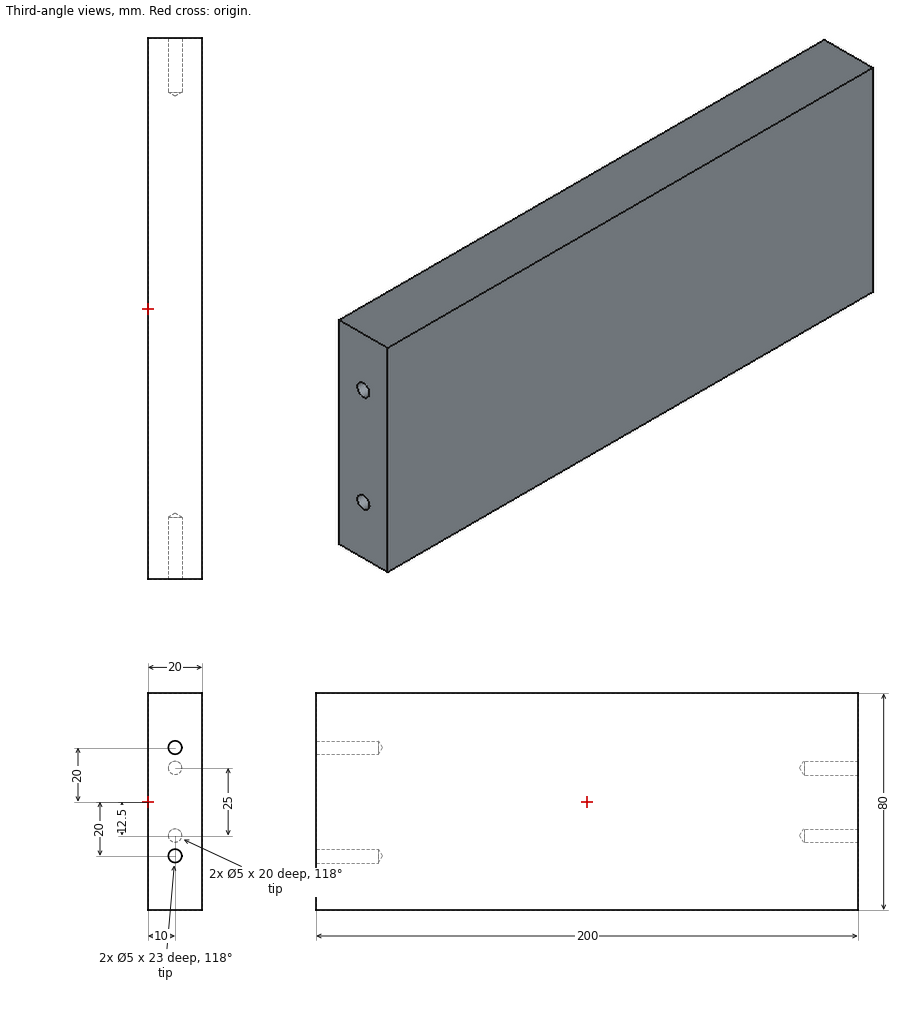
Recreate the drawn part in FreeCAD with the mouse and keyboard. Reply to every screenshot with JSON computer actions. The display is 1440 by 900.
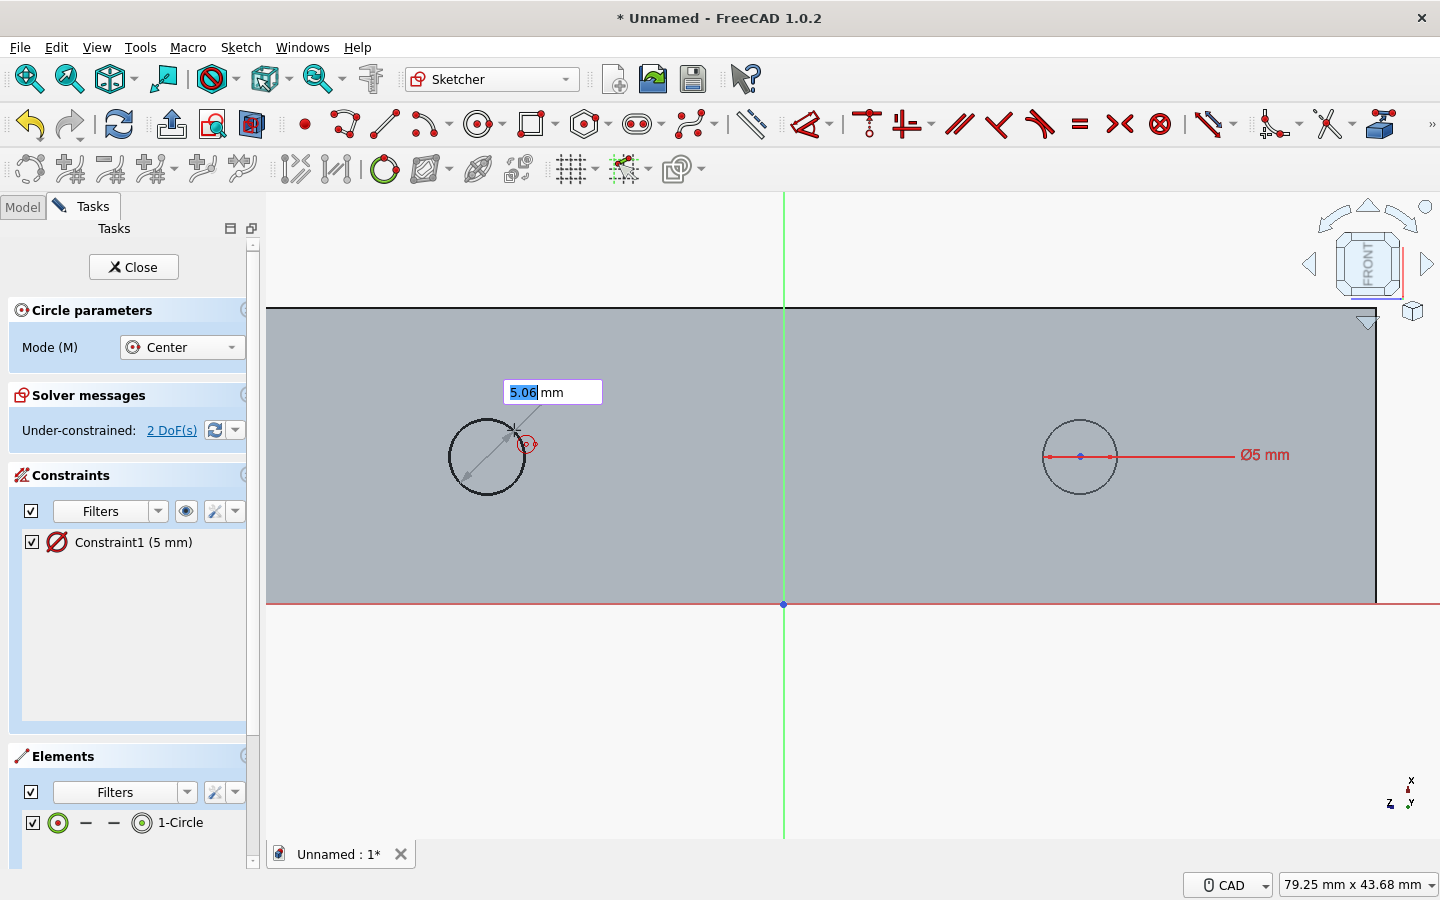
{"action": "type", "text": "5"}
{"action": "key", "text": "Return"}
{"action": "key", "text": "Escape"}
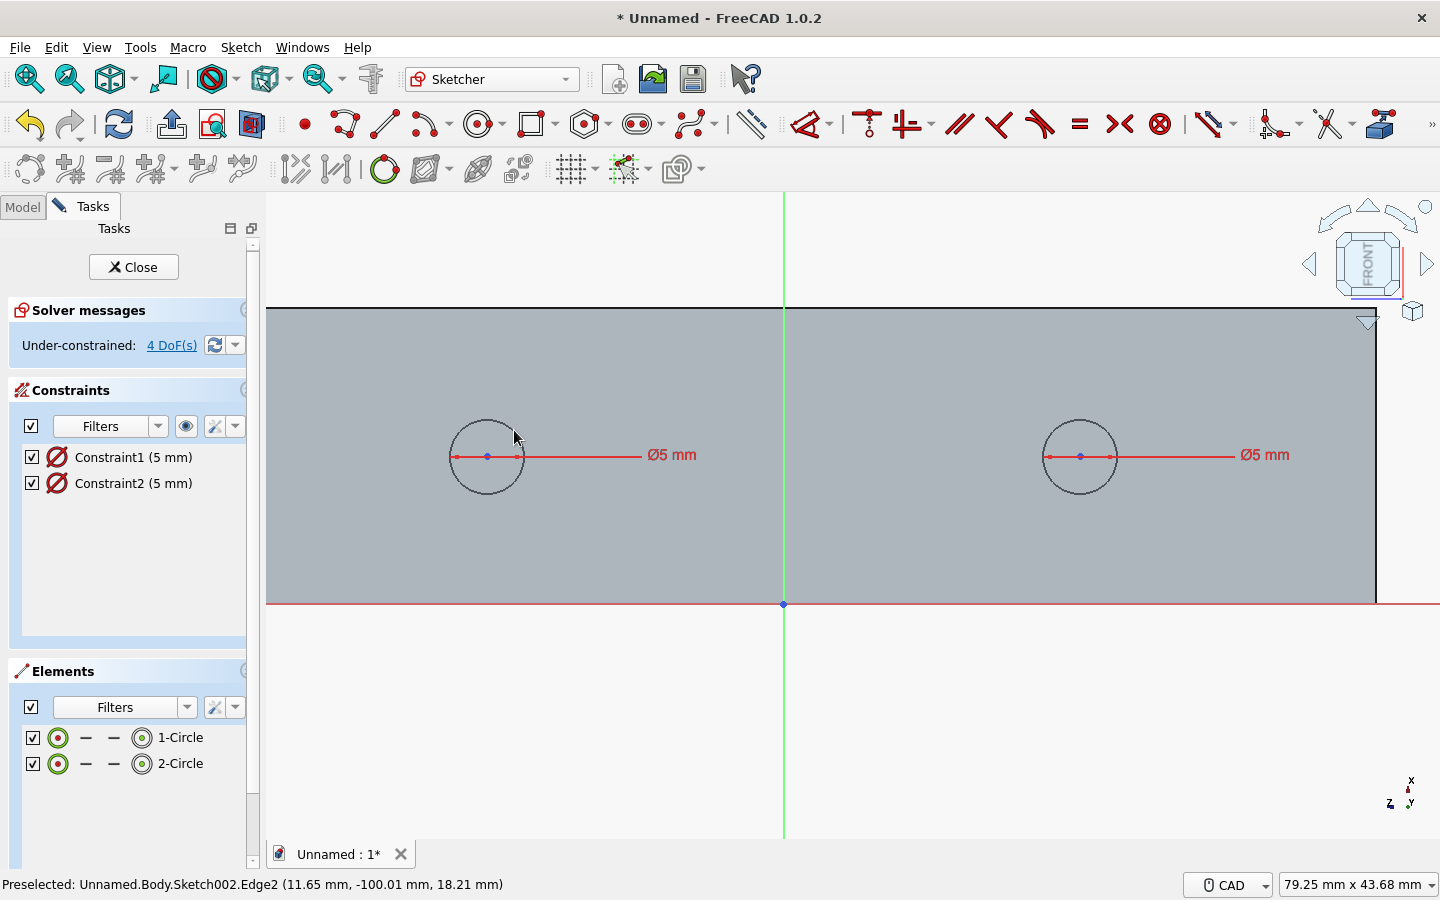
{"action": "left_click", "coordinate": [1080, 457]}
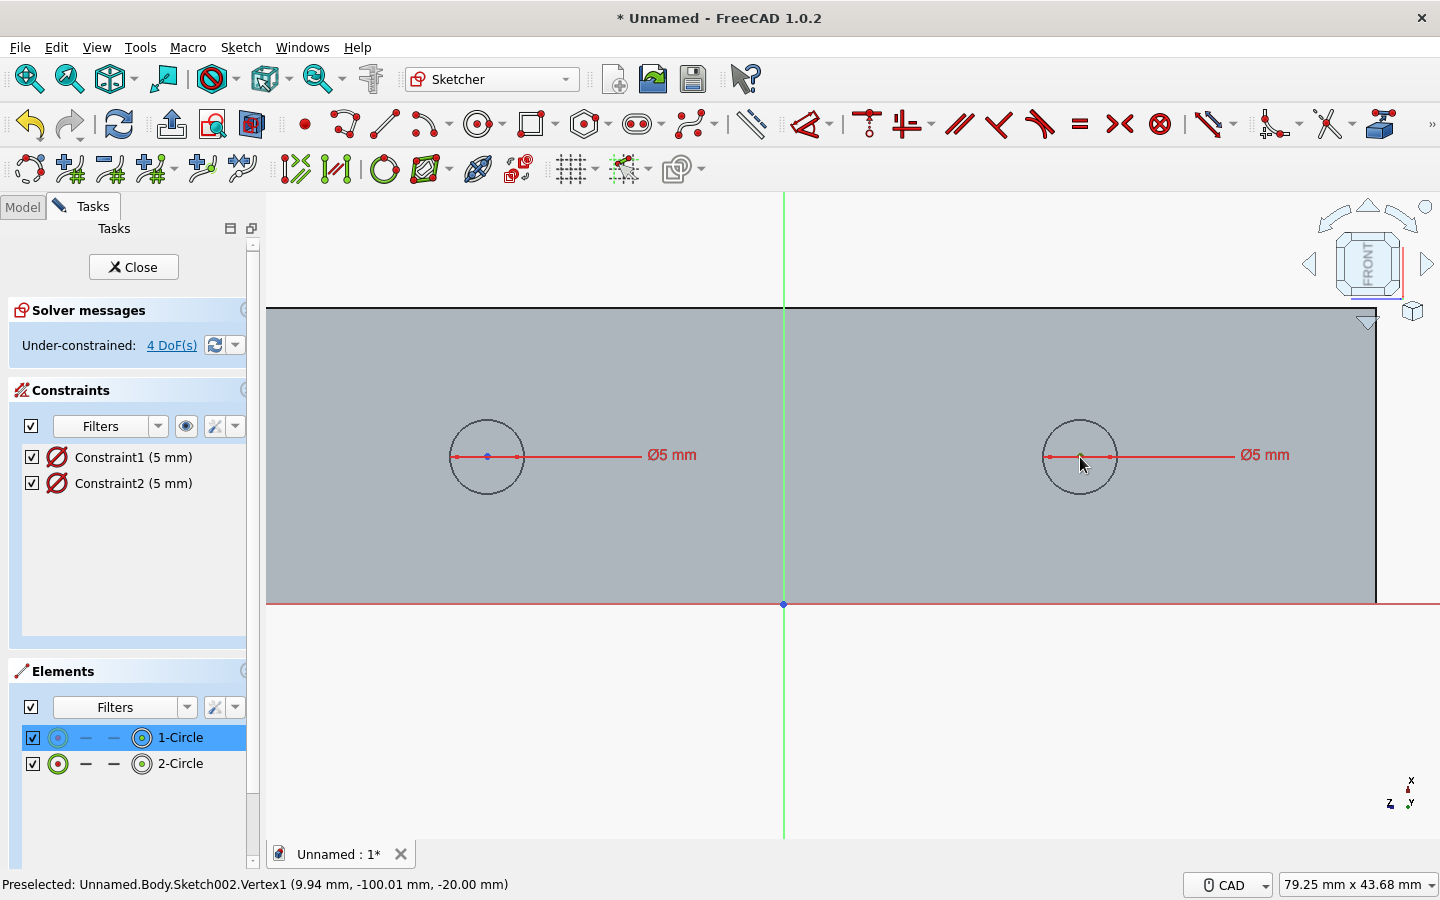
{"action": "left_click", "coordinate": [487, 457]}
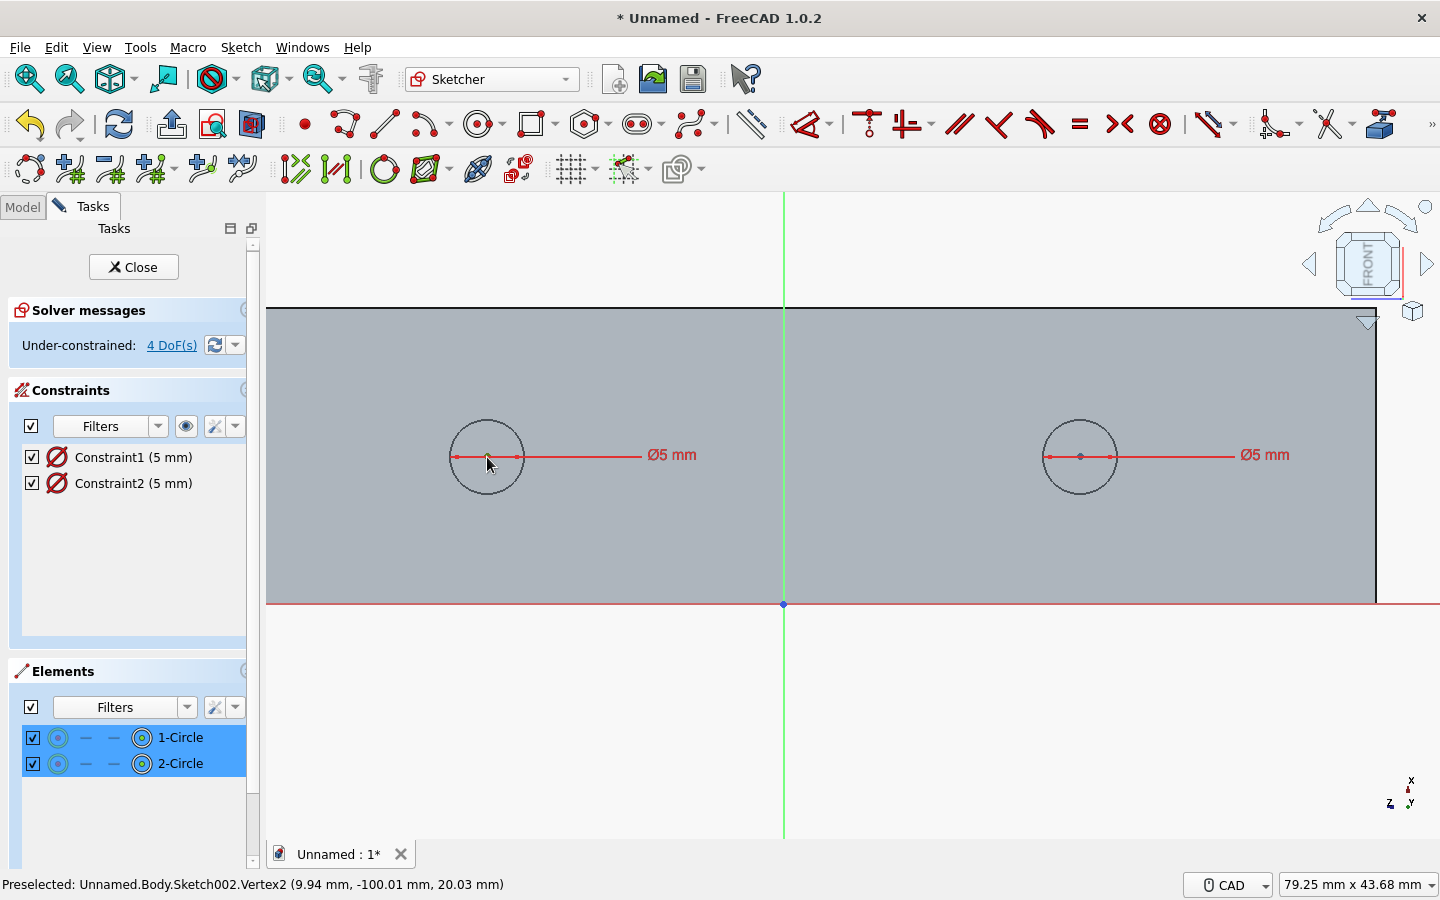
{"action": "key", "text": "h"}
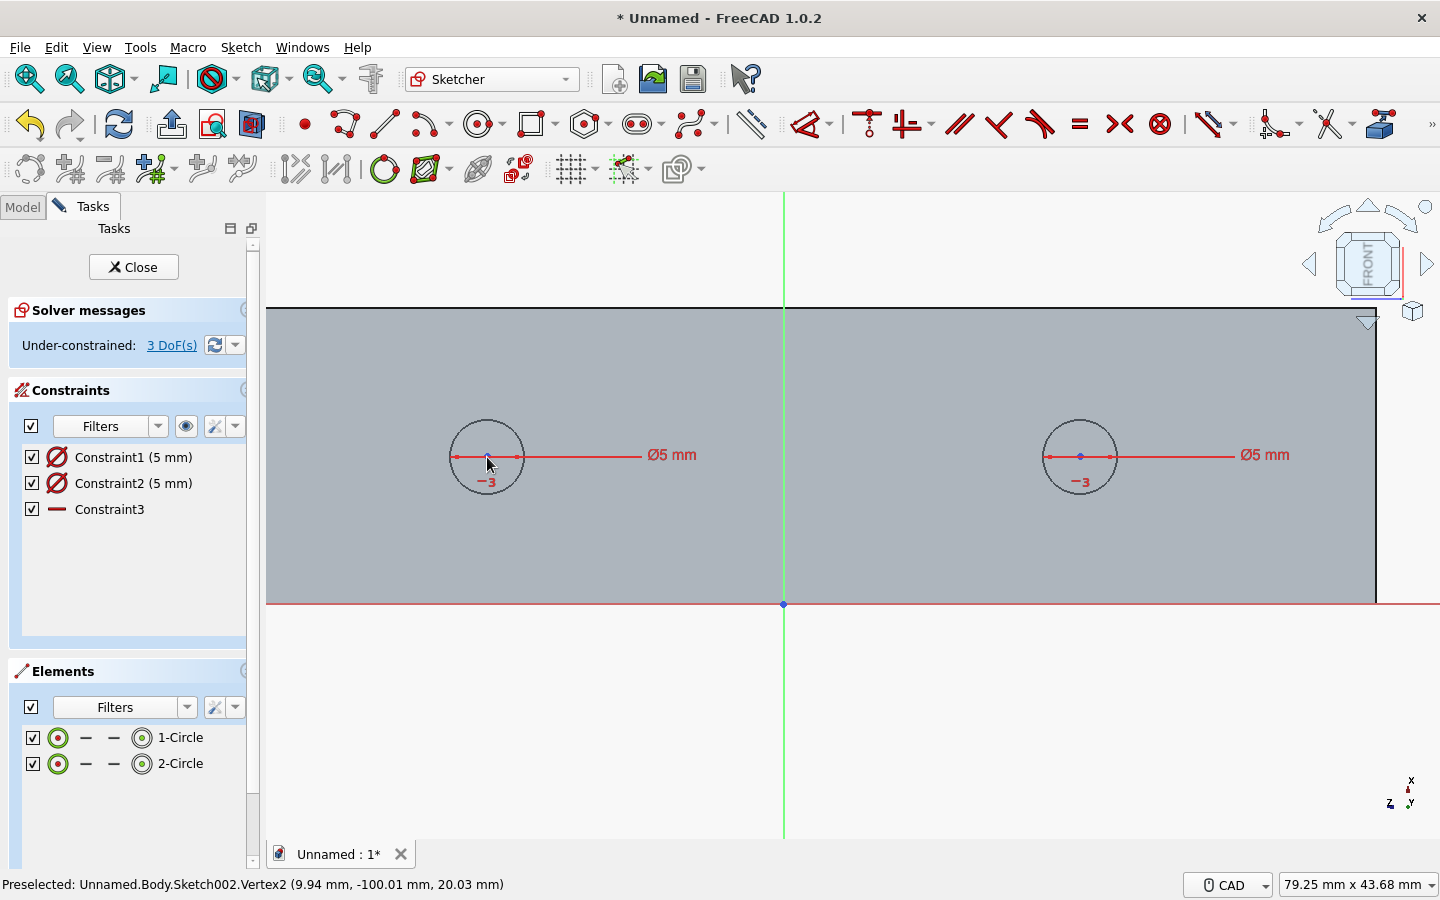
{"action": "left_click", "coordinate": [806, 124]}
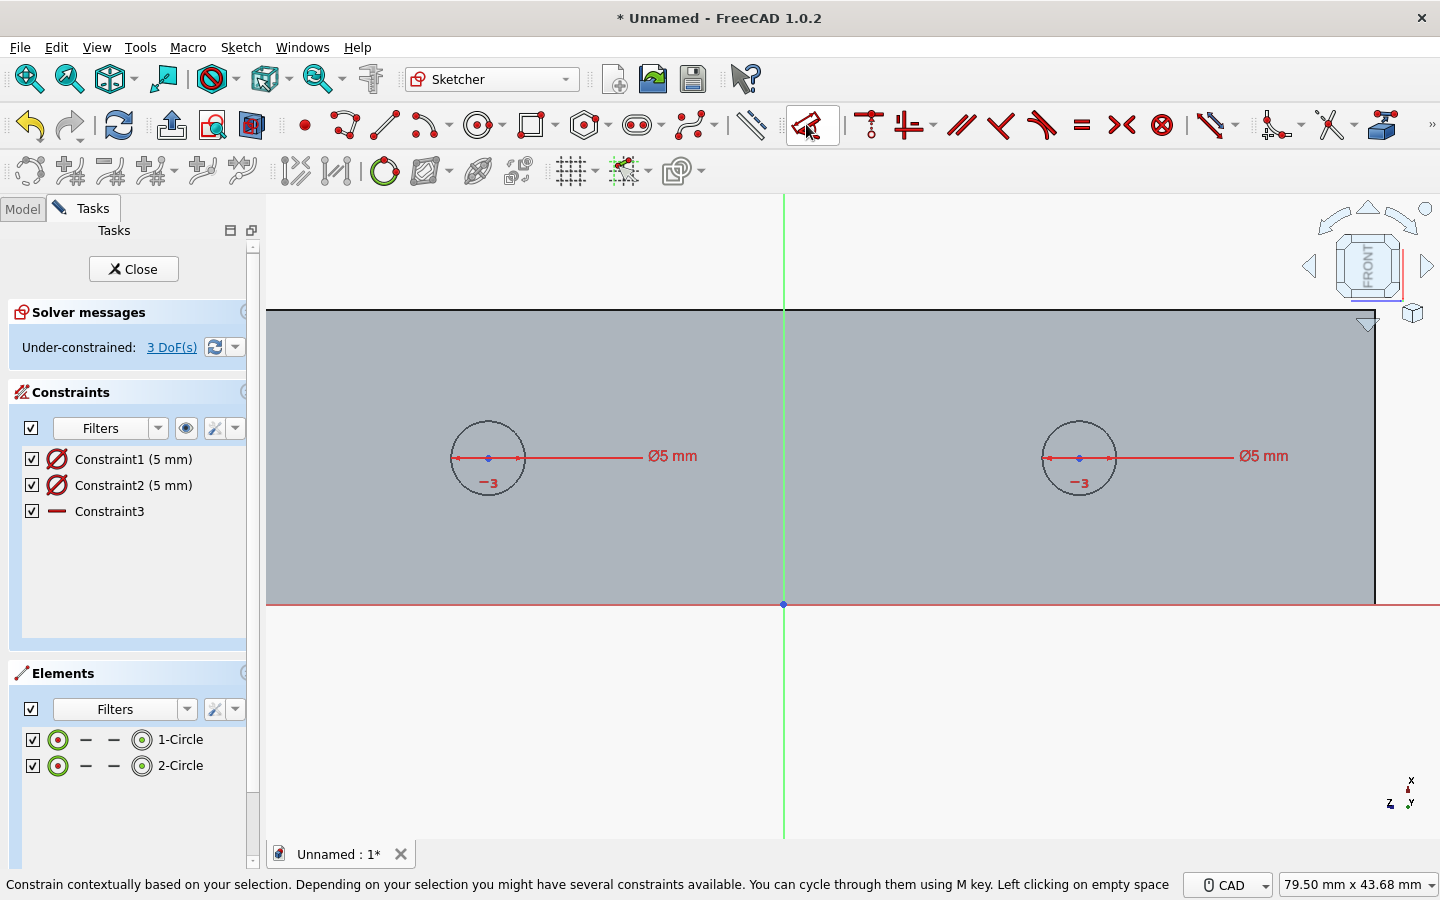
{"action": "left_click", "coordinate": [1079, 458]}
{"action": "left_click", "coordinate": [932, 639]}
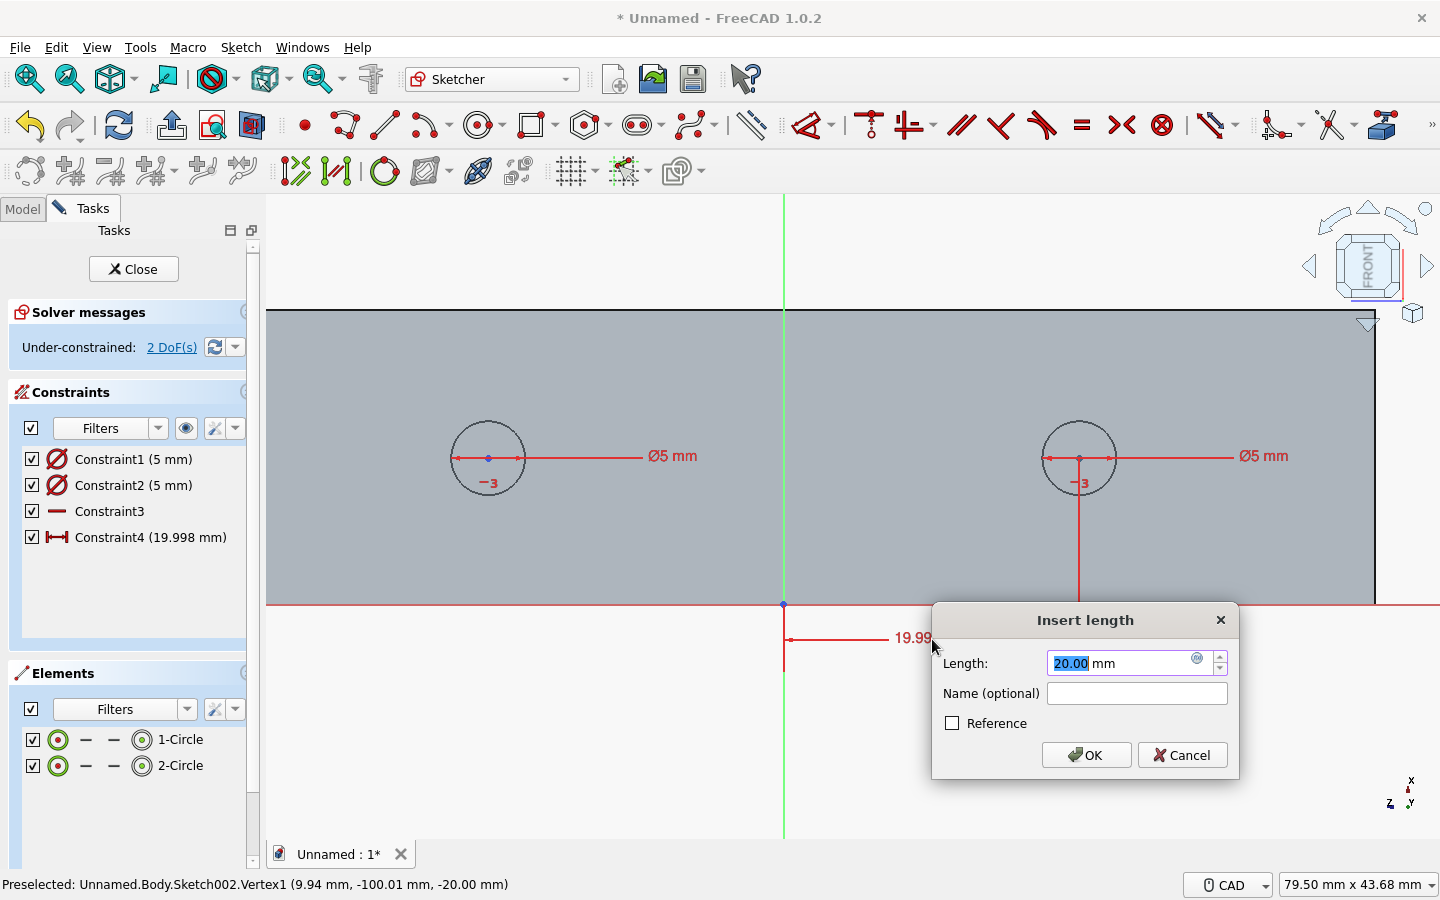
{"action": "type", "text": "20"}
{"action": "key", "text": "Return"}